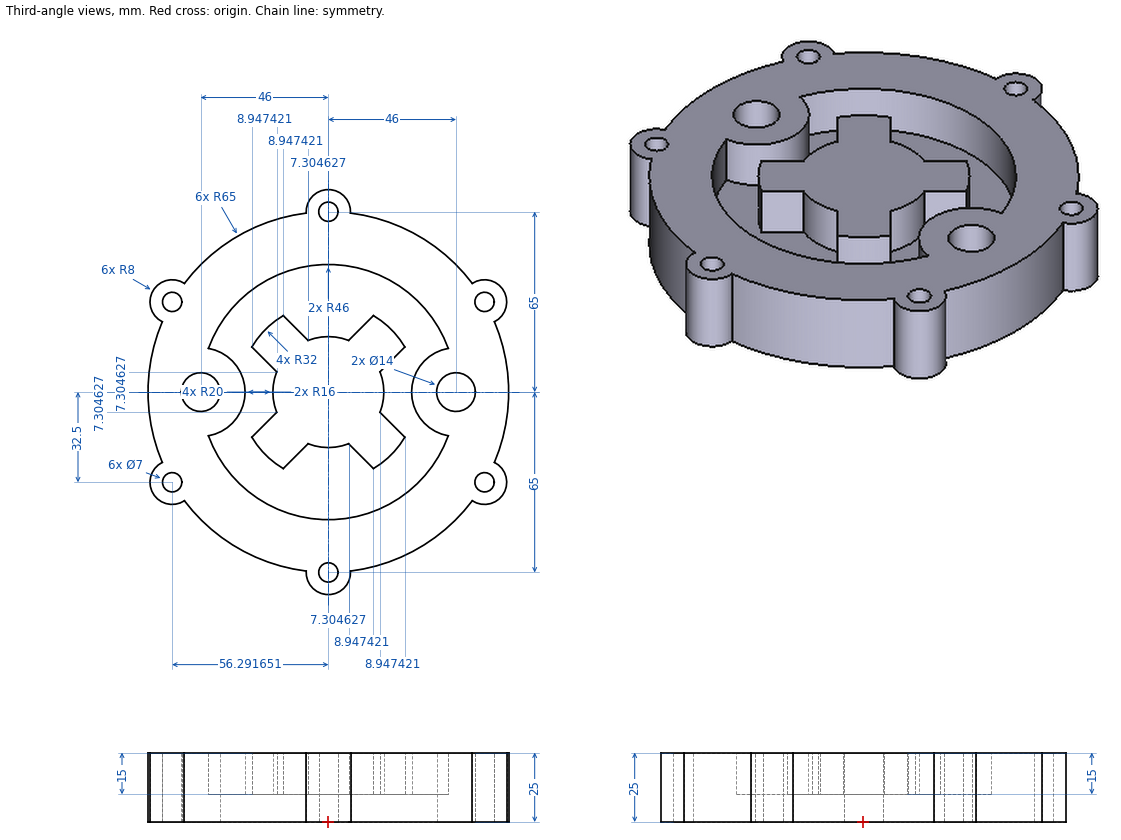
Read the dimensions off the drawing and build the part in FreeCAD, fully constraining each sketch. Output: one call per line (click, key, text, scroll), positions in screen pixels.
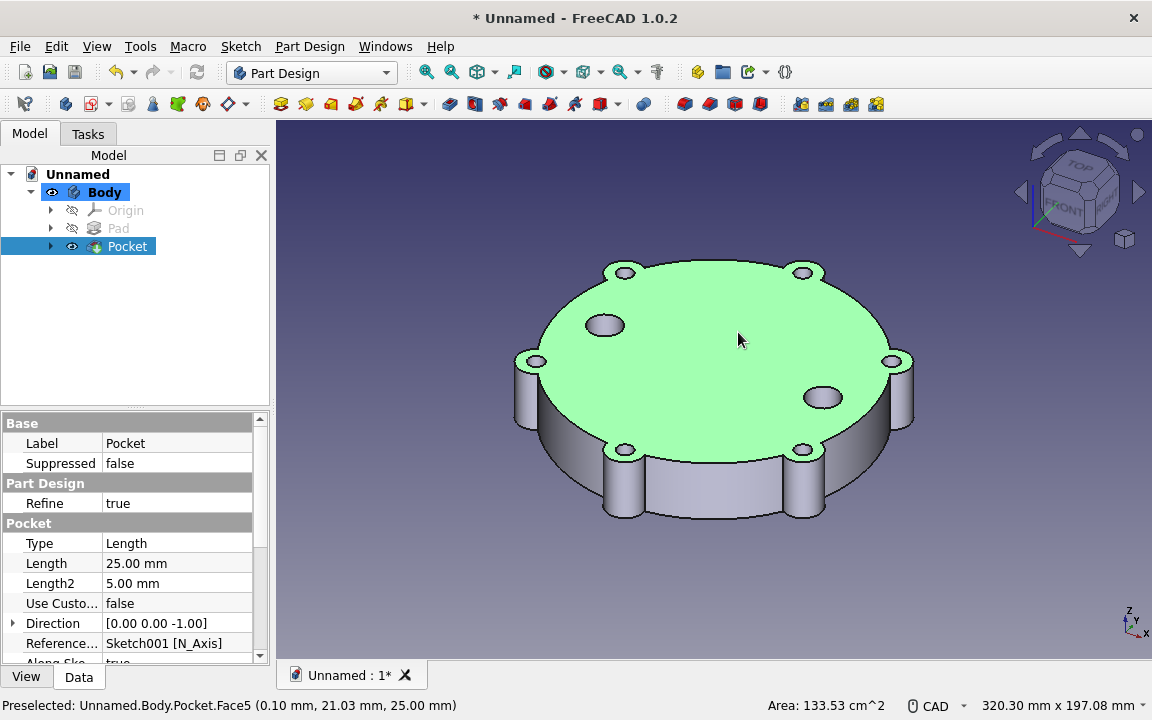
click(90, 104)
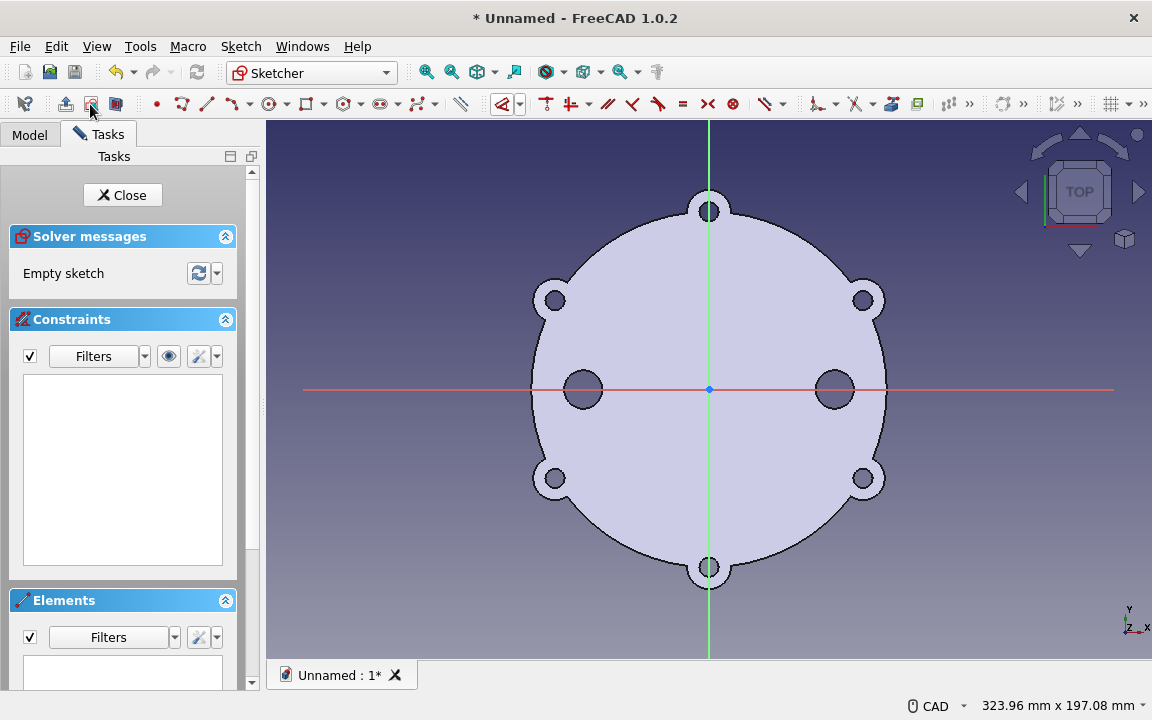
scroll(848, 390, up, 2)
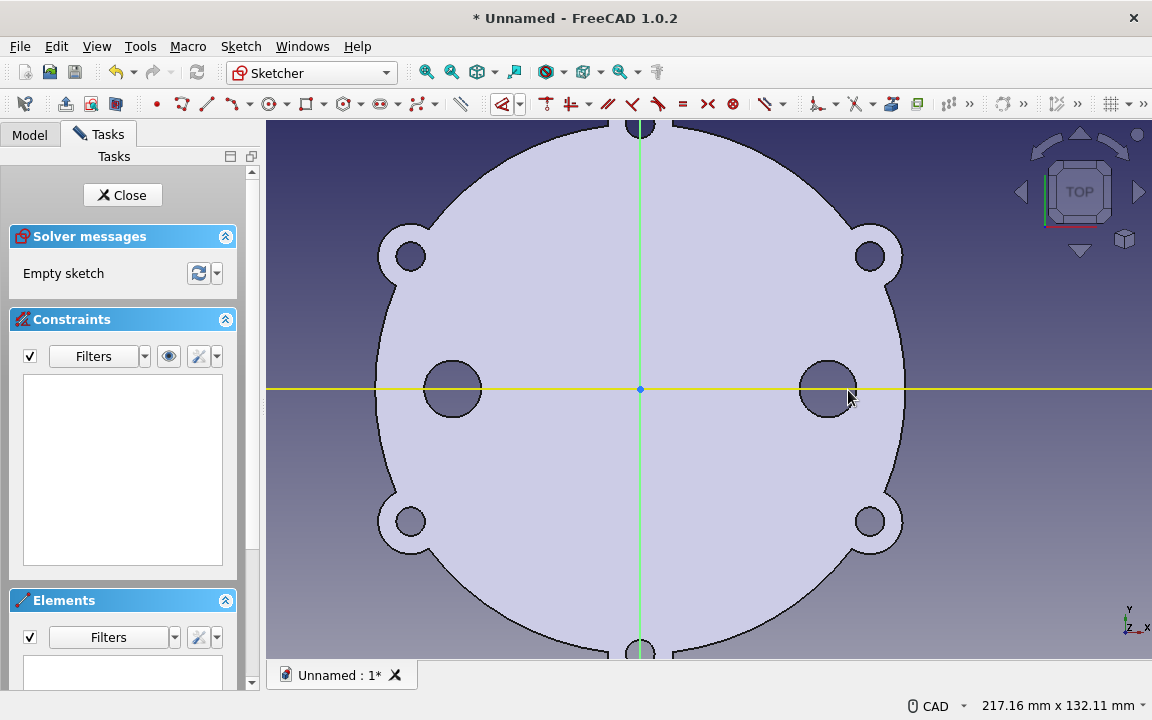
click(232, 104)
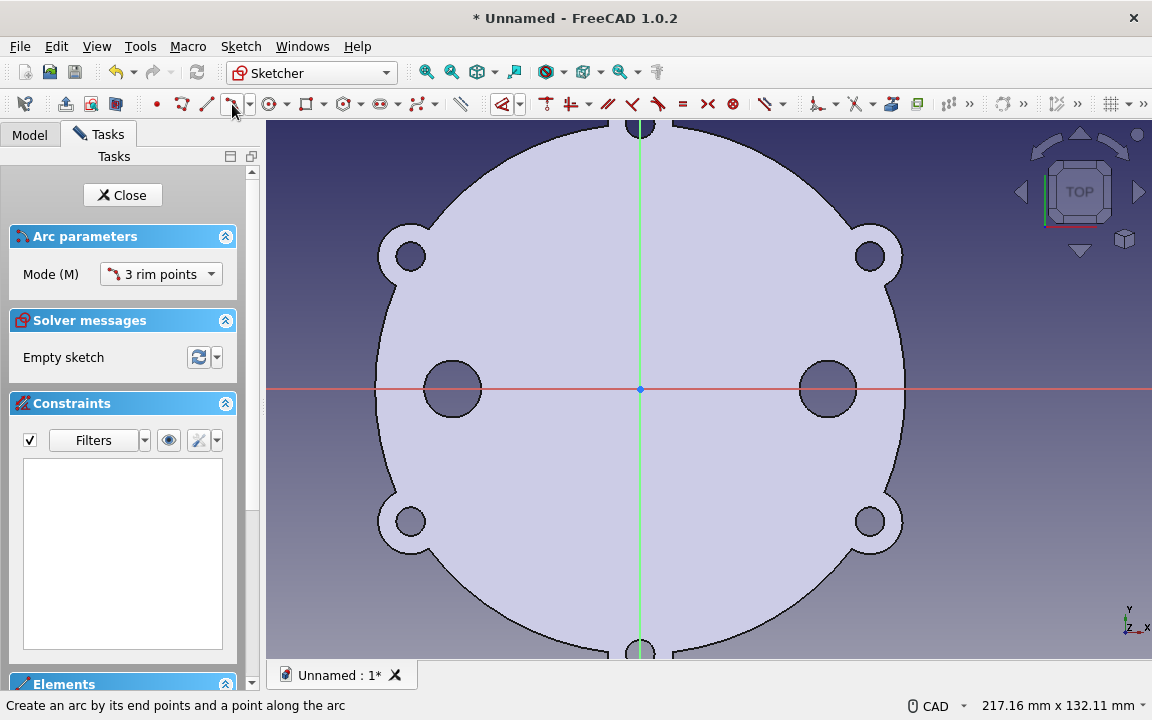
click(817, 325)
click(464, 325)
click(686, 207)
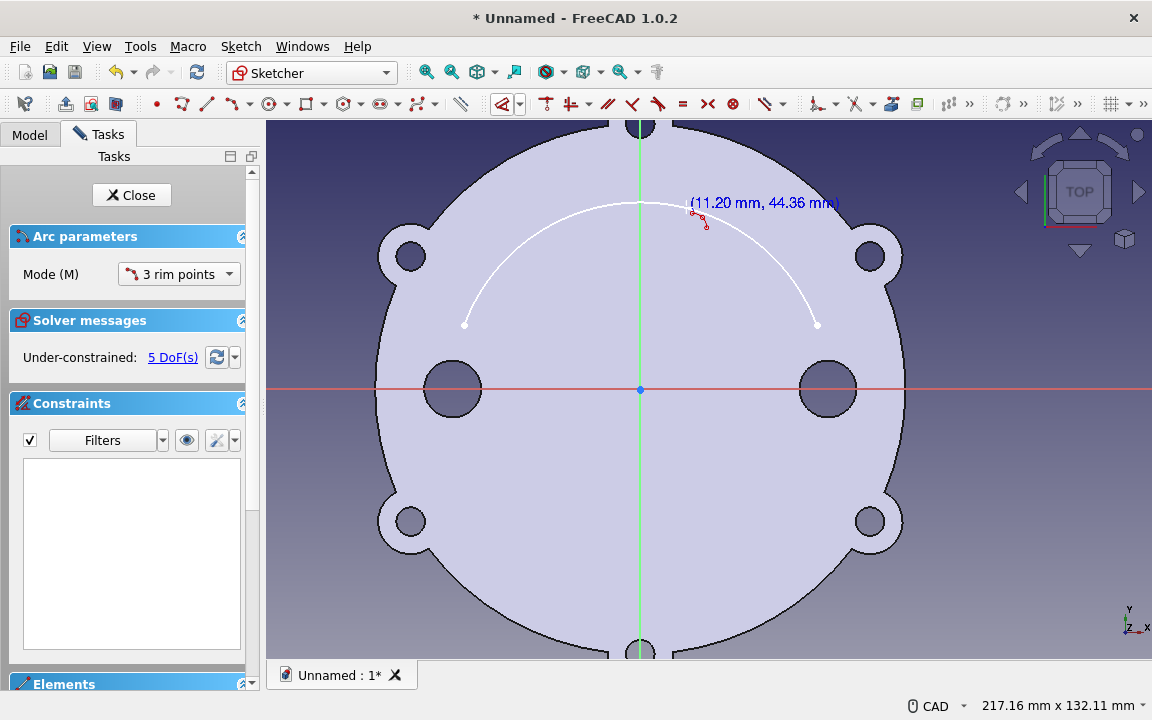
click(464, 326)
click(464, 453)
click(515, 407)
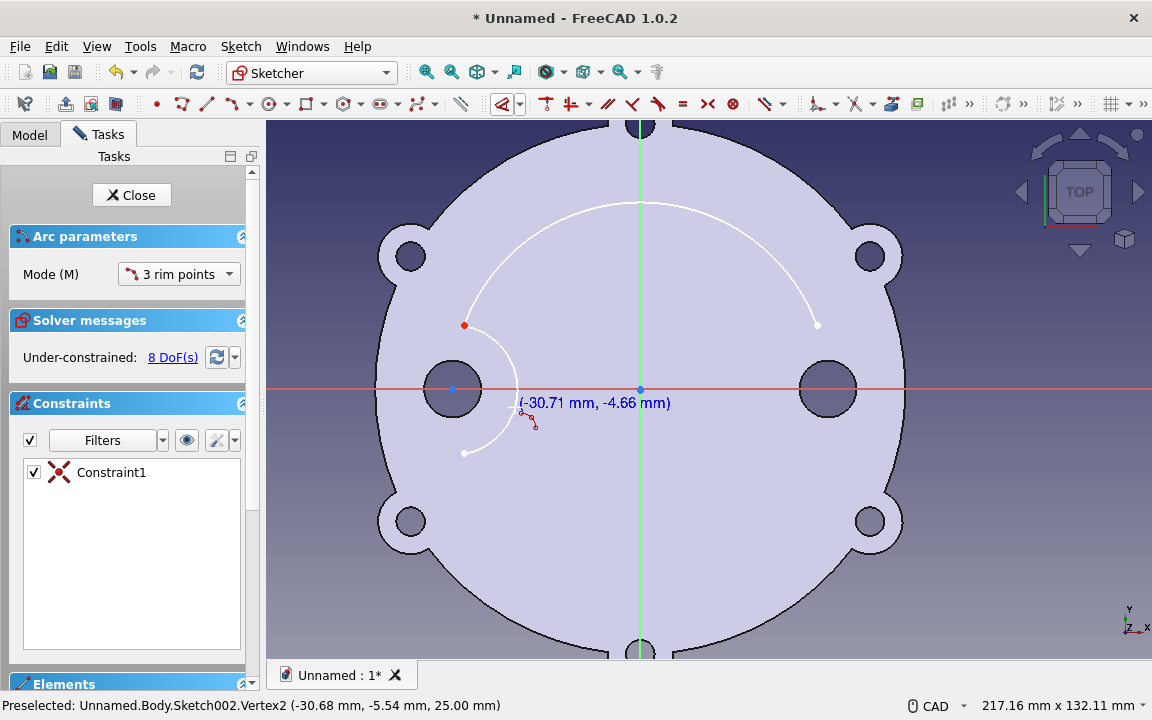
click(464, 454)
click(817, 453)
click(595, 571)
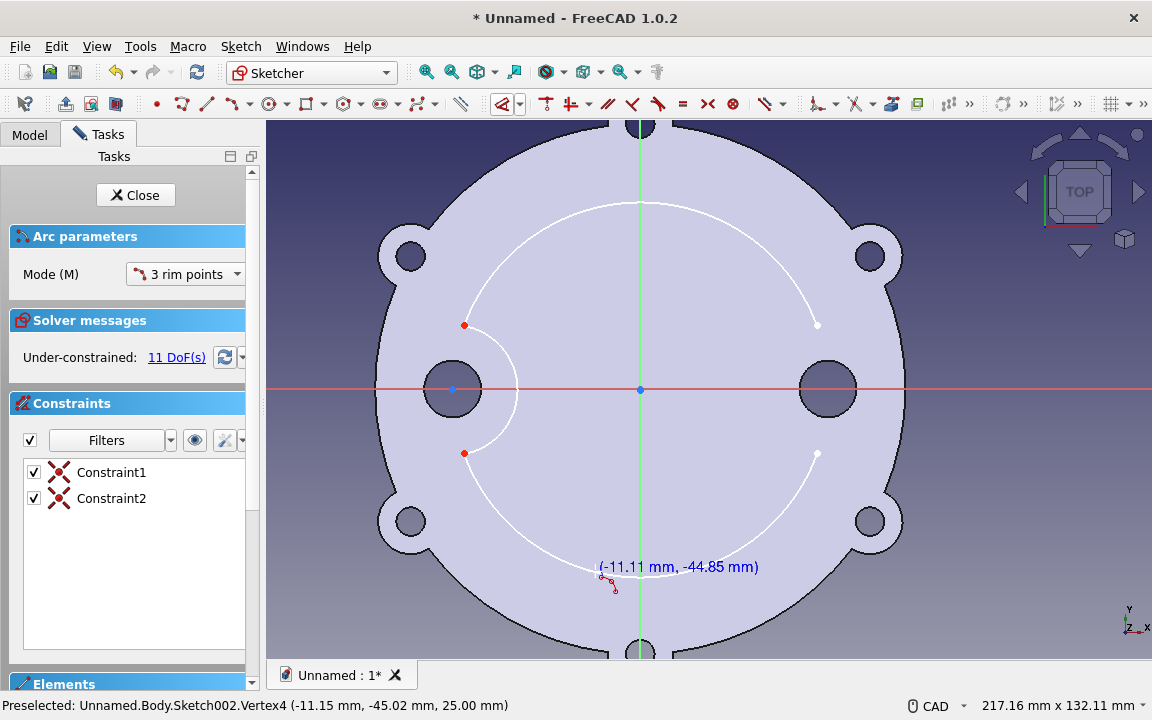
click(817, 454)
click(817, 326)
click(765, 371)
key(Escape)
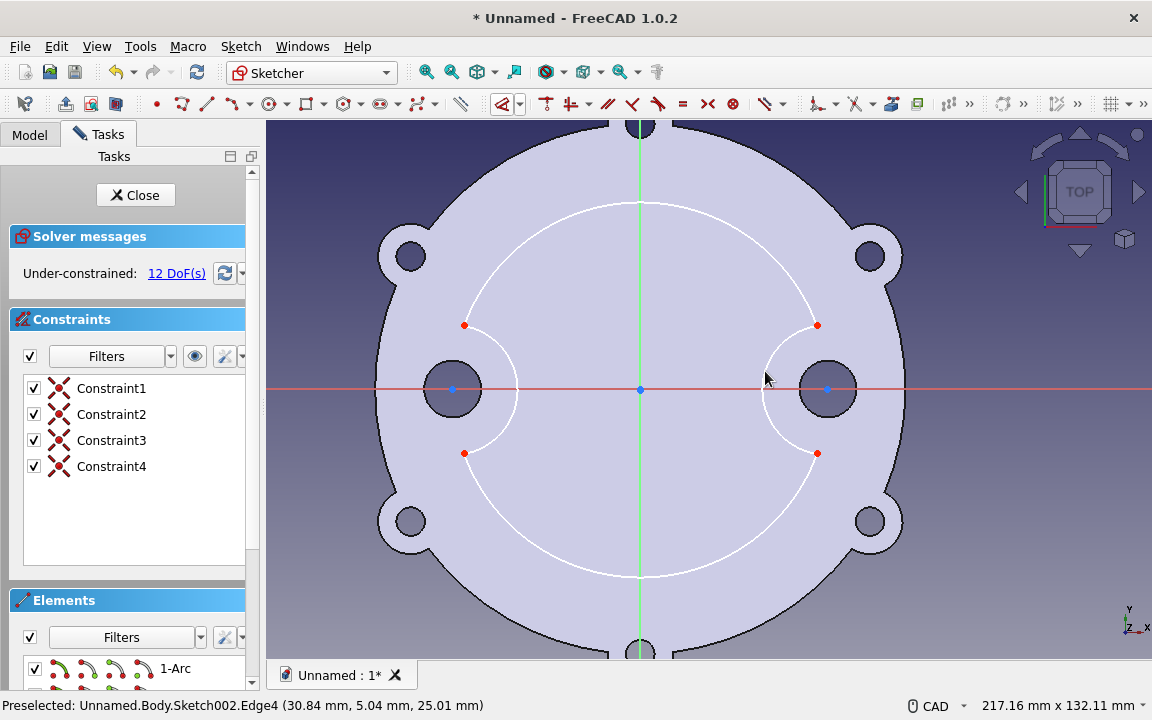
click(729, 224)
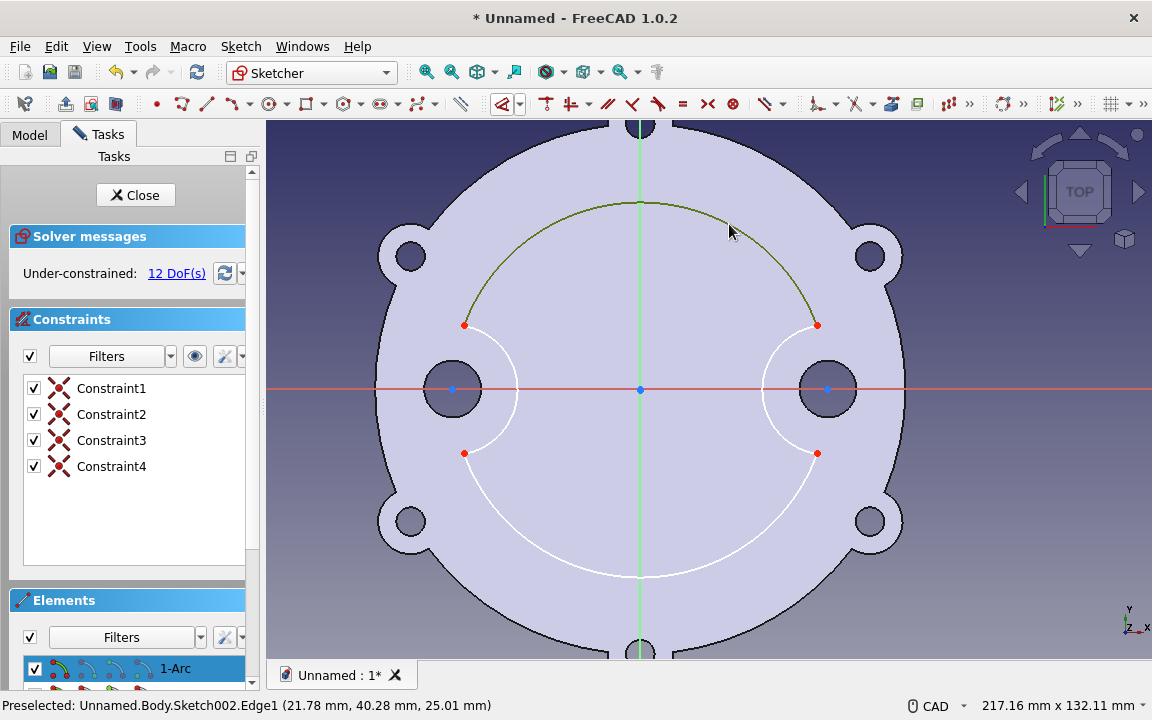
click(552, 556)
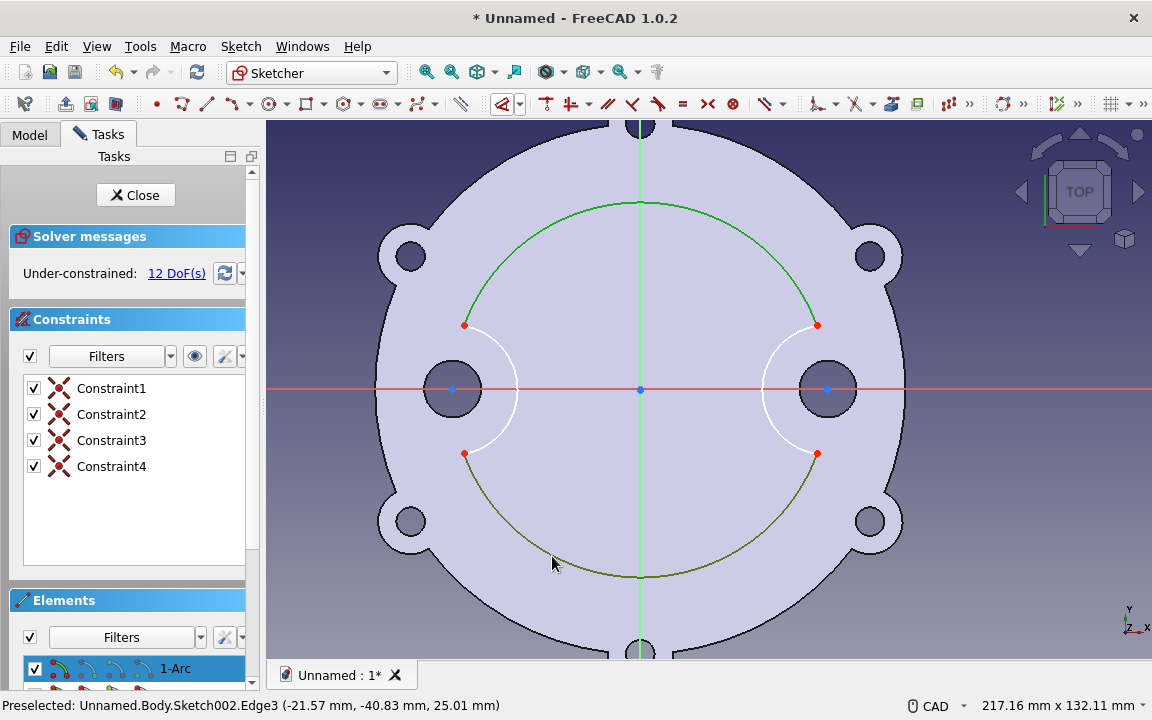
click(546, 104)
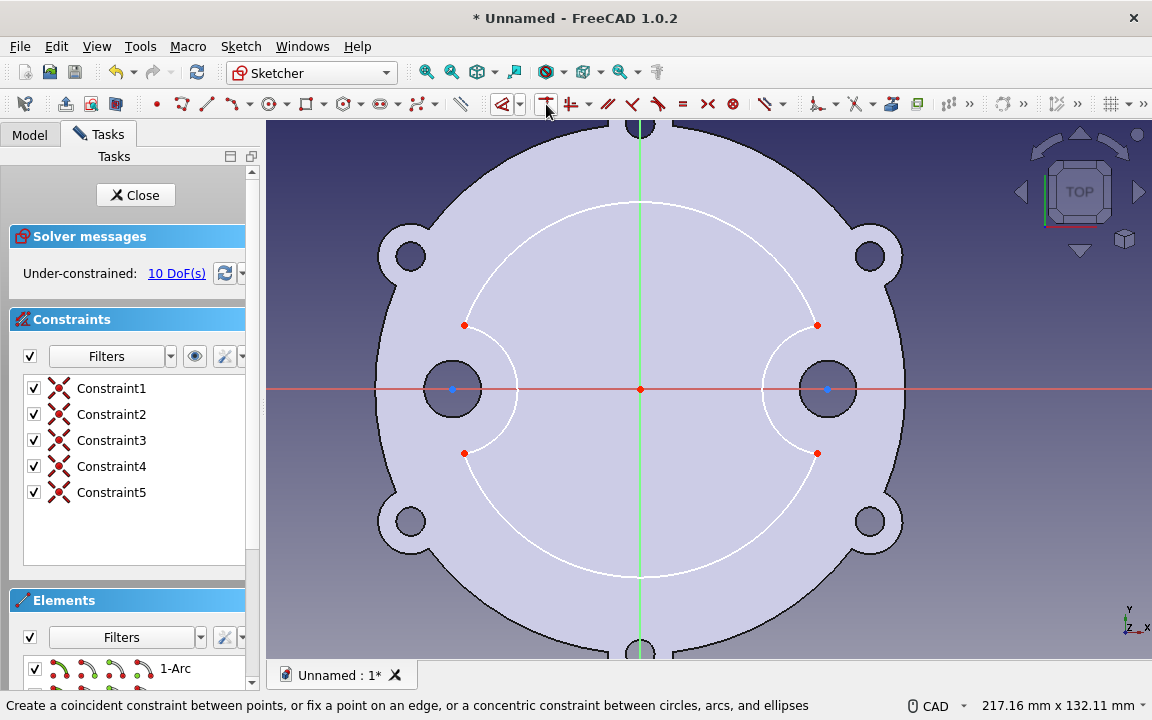
drag(630, 379, 650, 400)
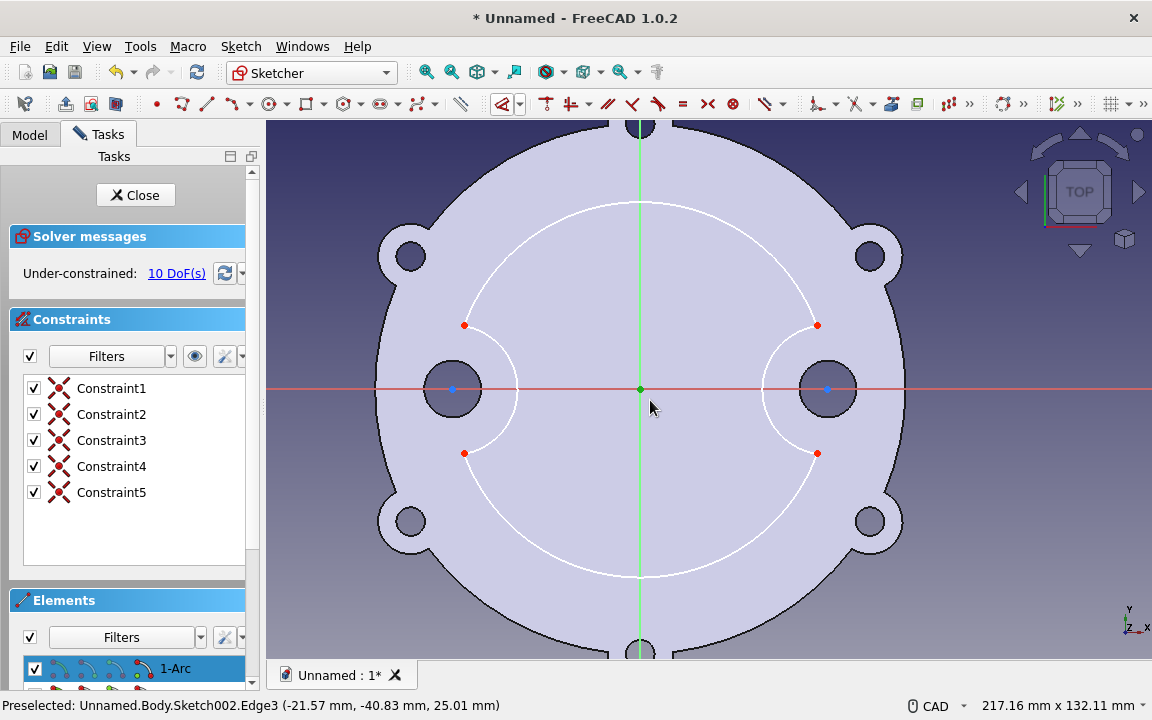
click(546, 104)